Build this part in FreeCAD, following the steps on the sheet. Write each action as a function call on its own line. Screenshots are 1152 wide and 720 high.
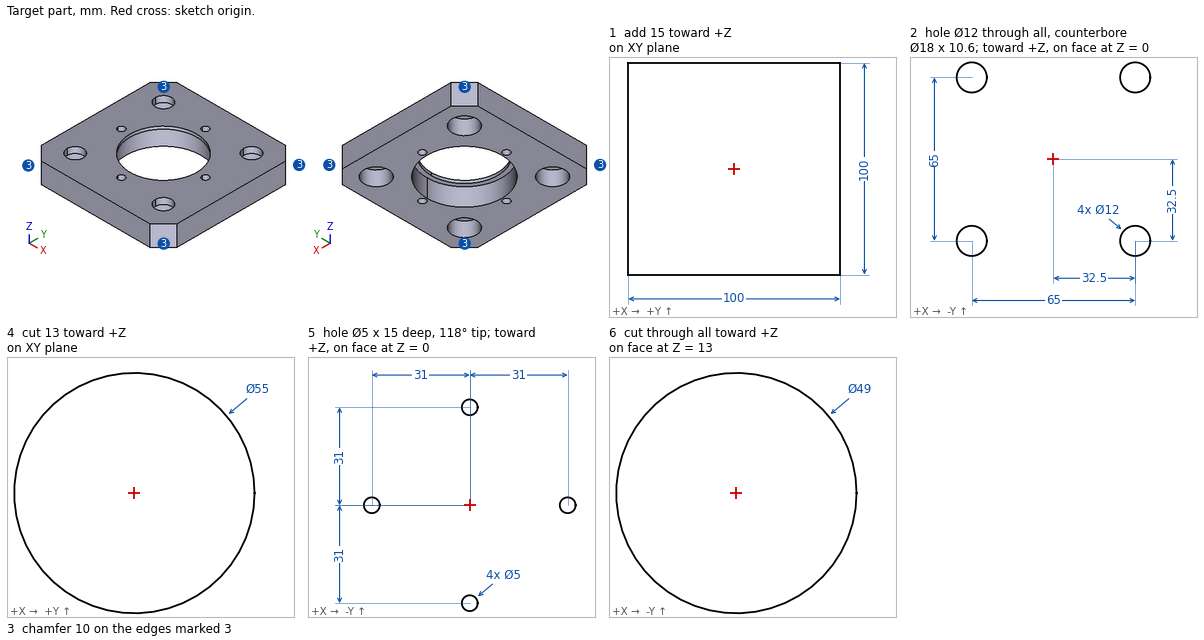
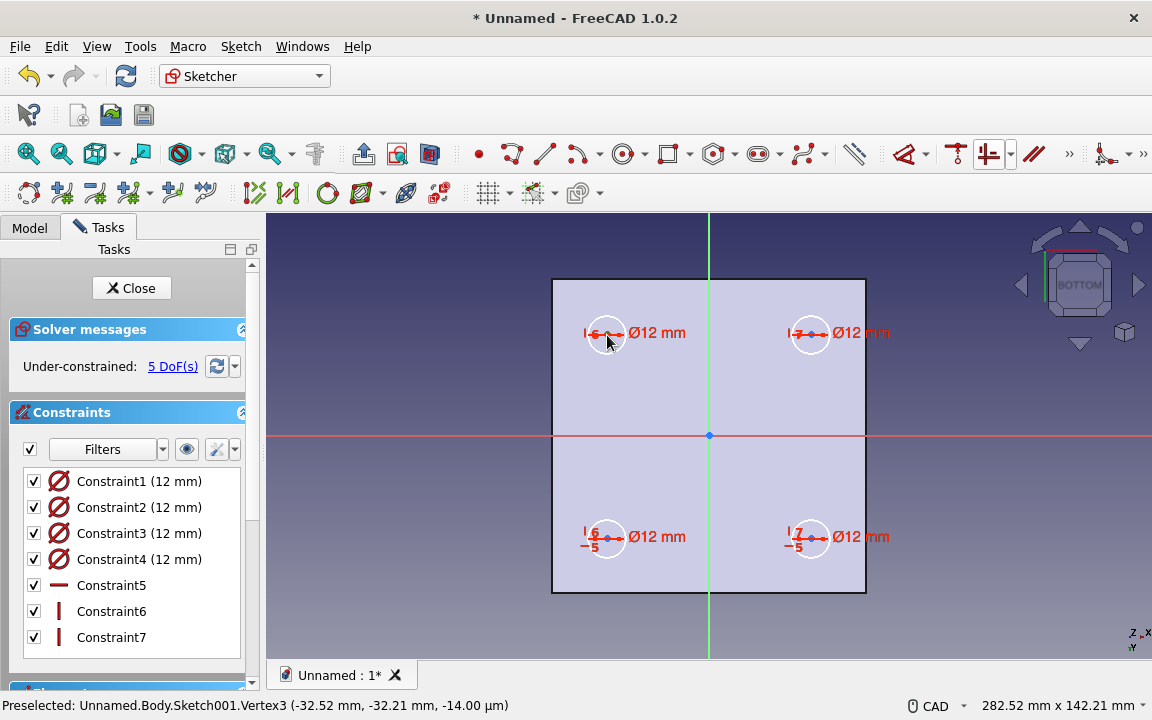
click(811, 335)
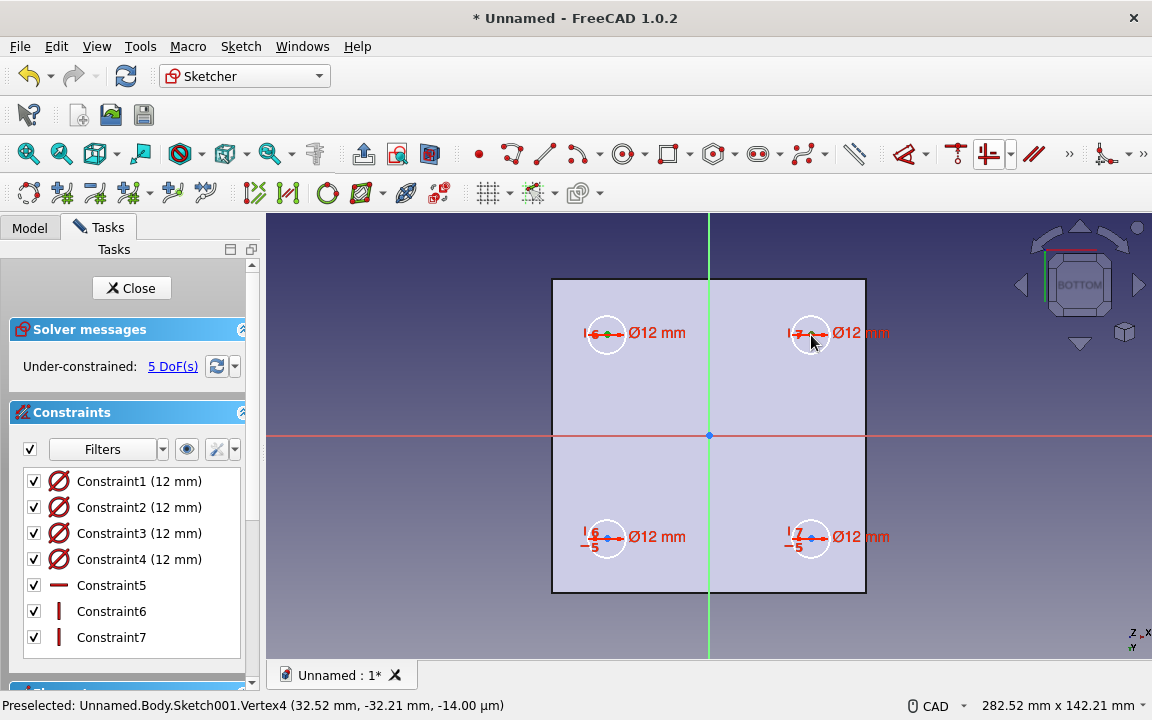
click(1010, 154)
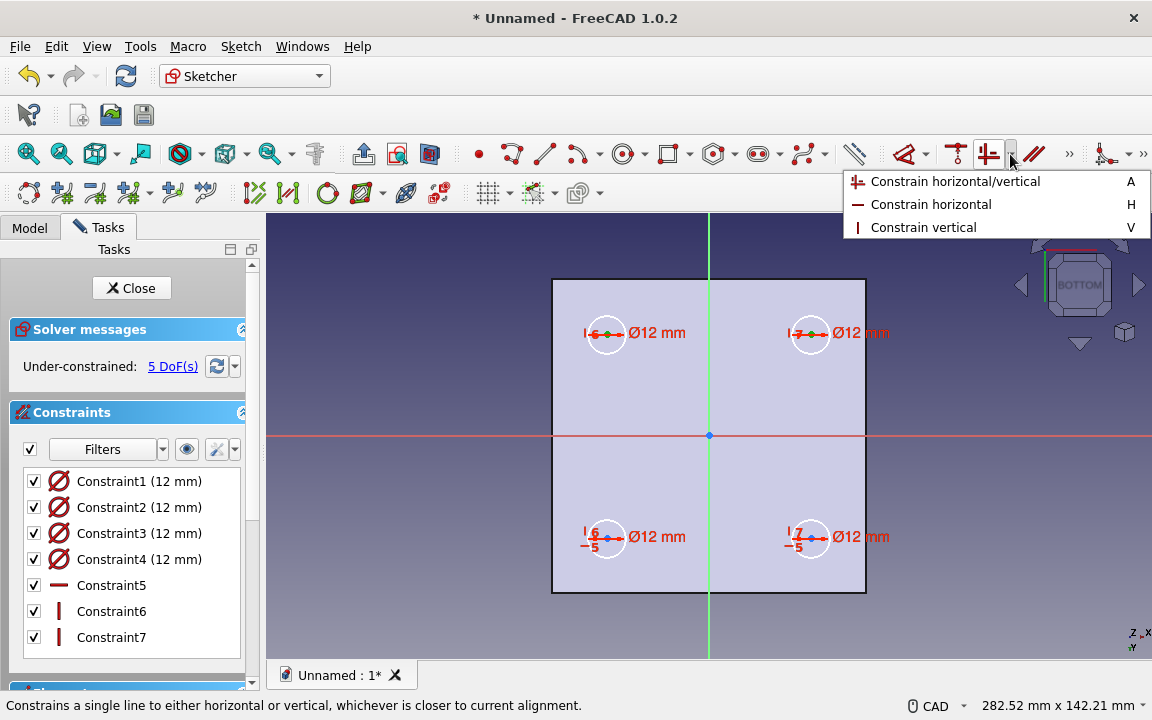
click(997, 204)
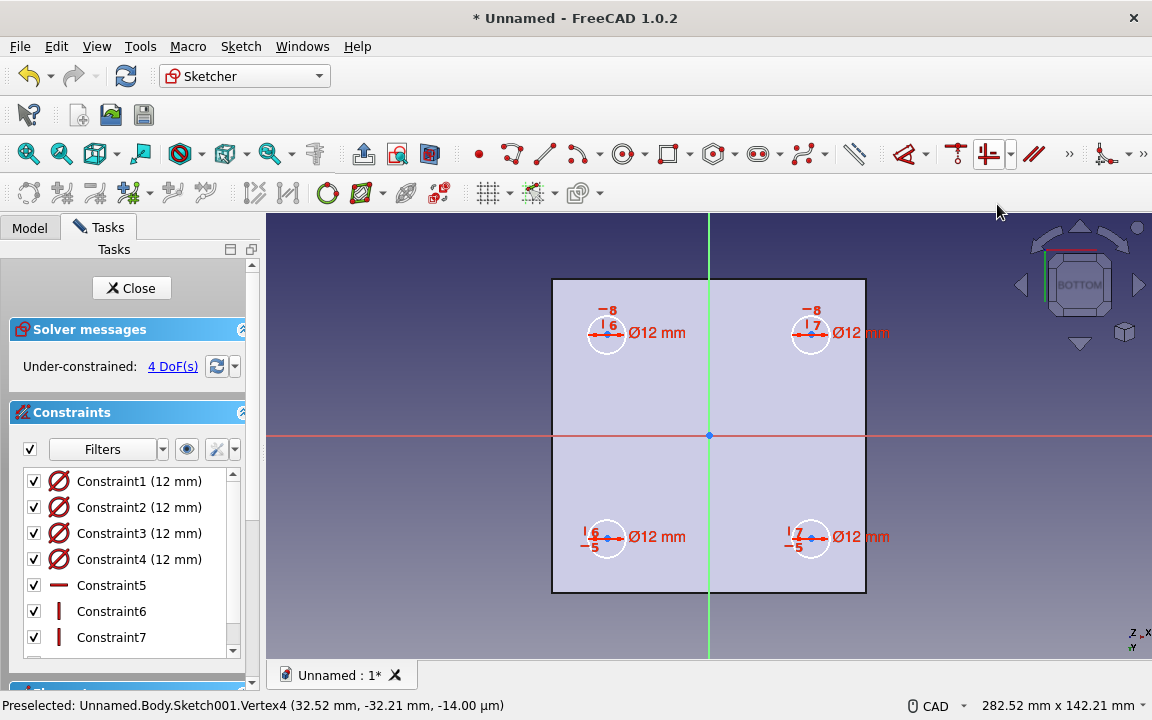
click(904, 154)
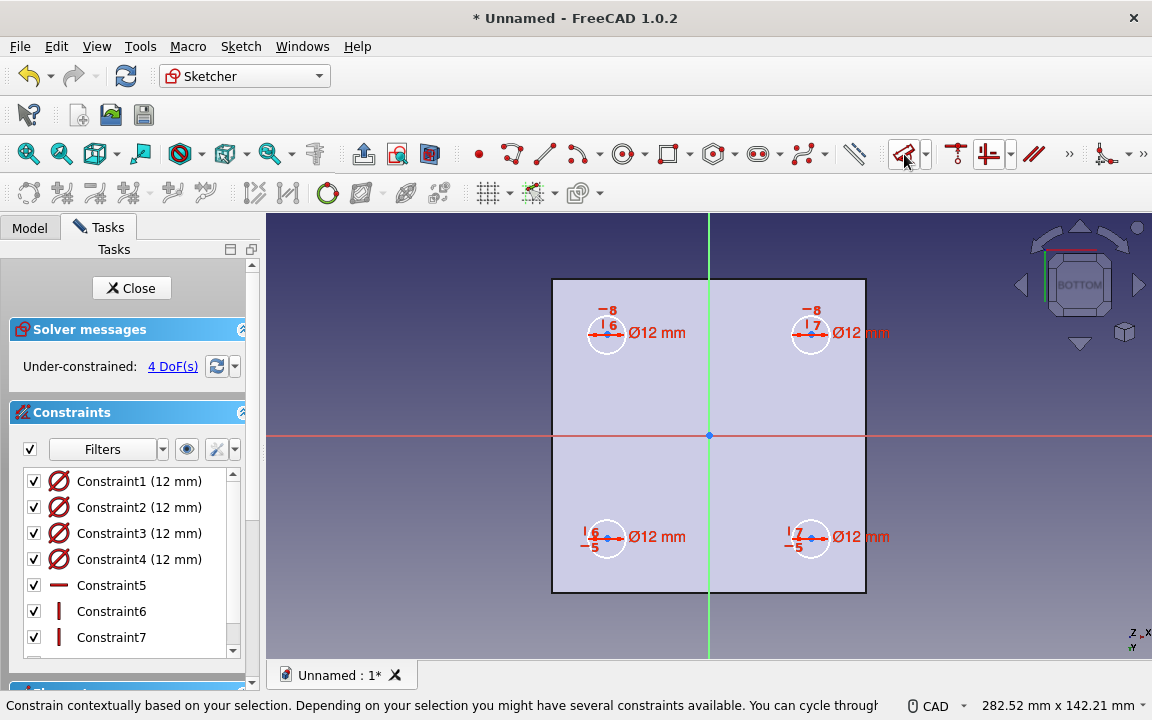
click(811, 539)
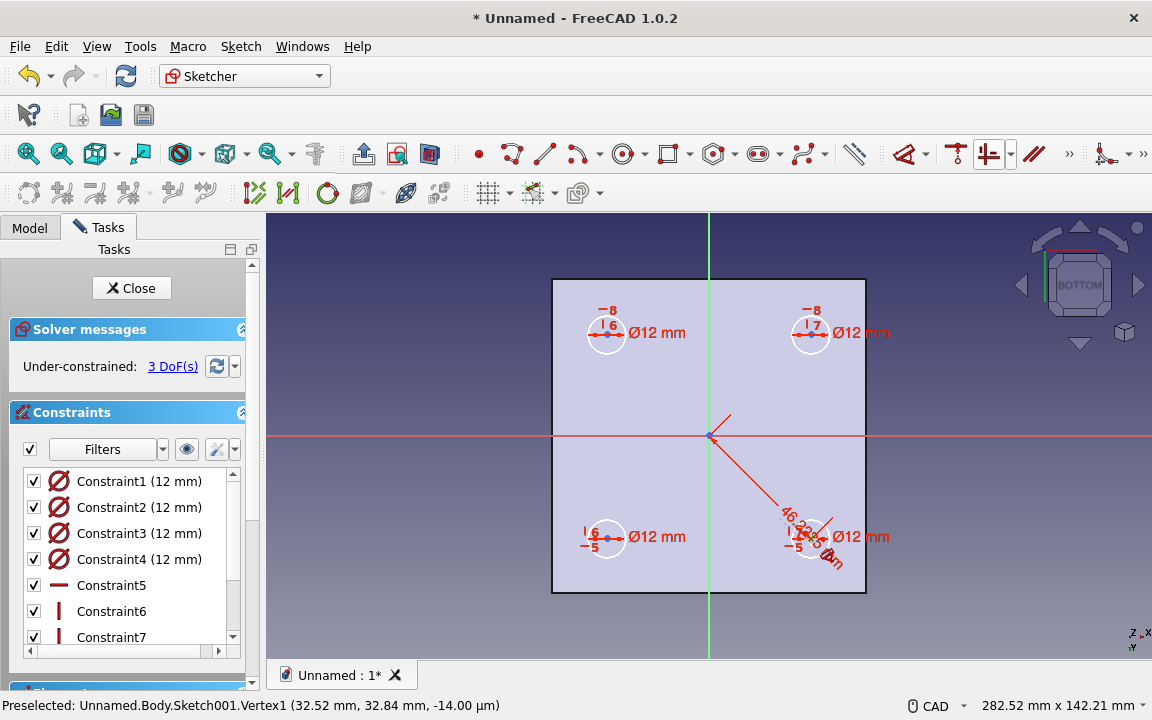
click(607, 539)
click(662, 573)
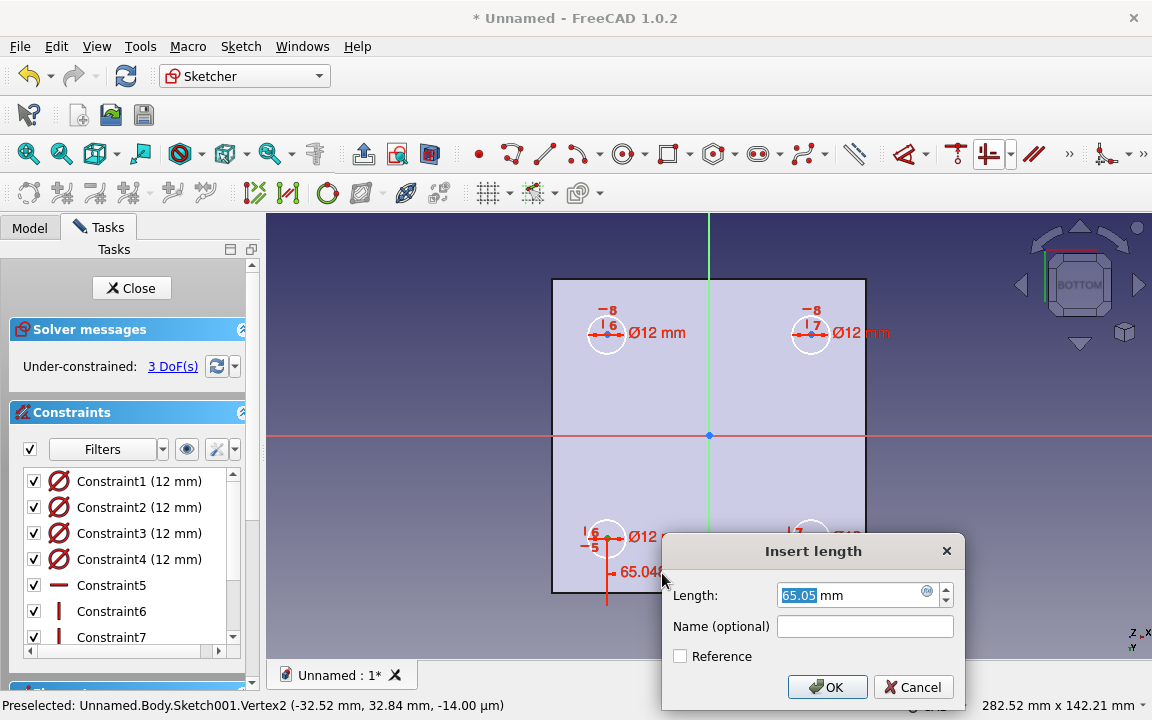
text(65)
key(Return)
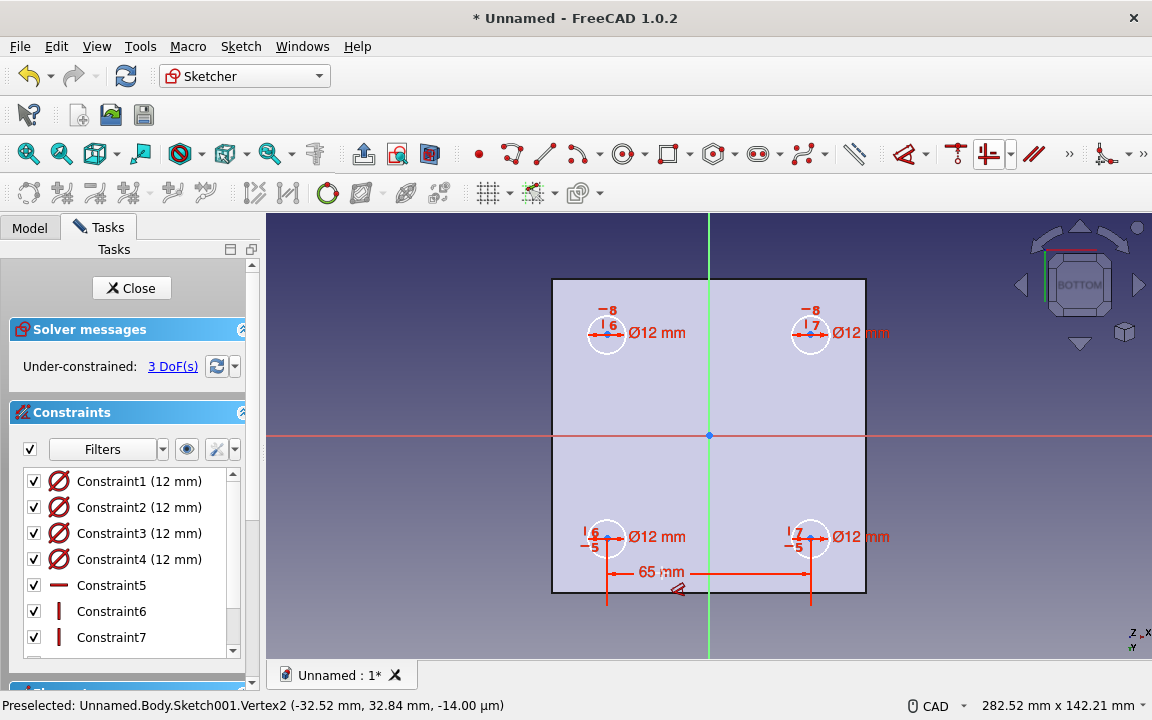
click(607, 539)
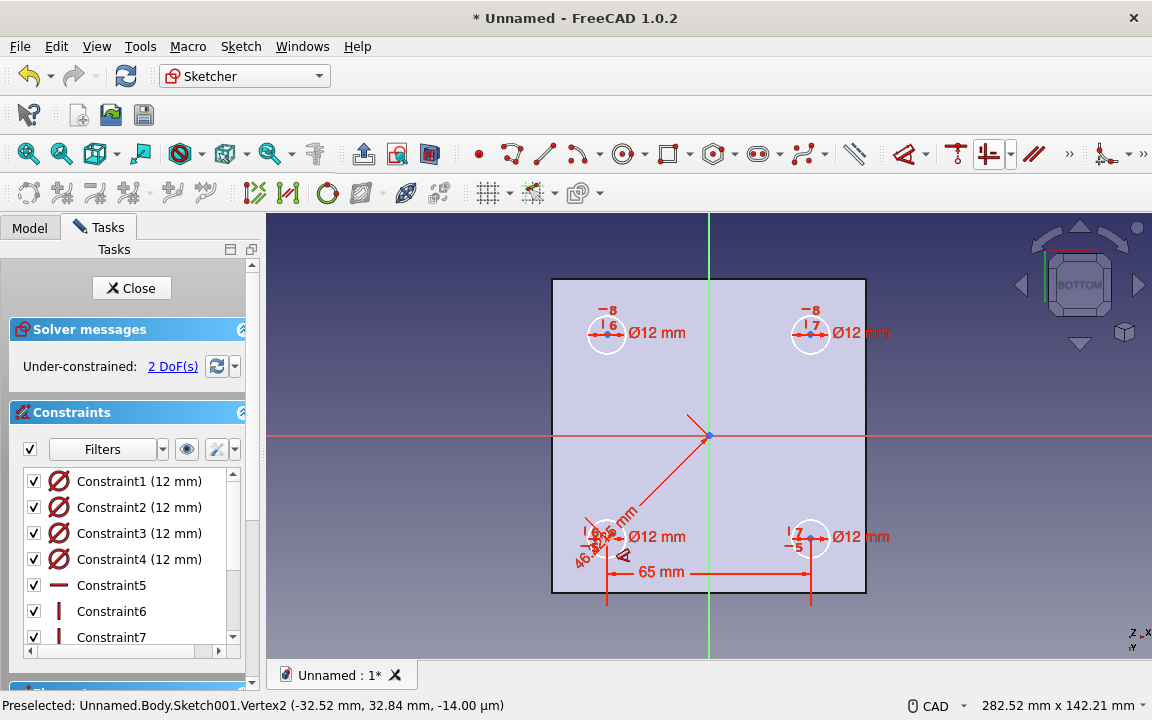
click(607, 335)
click(573, 390)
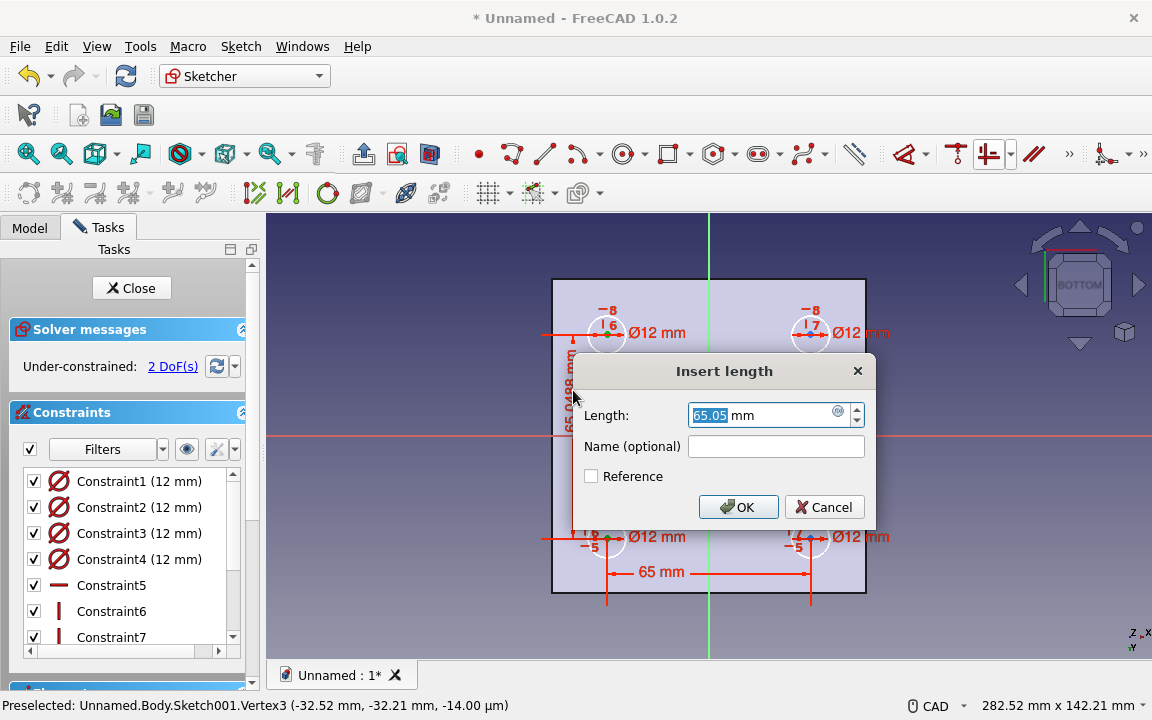
text(65)
key(Return)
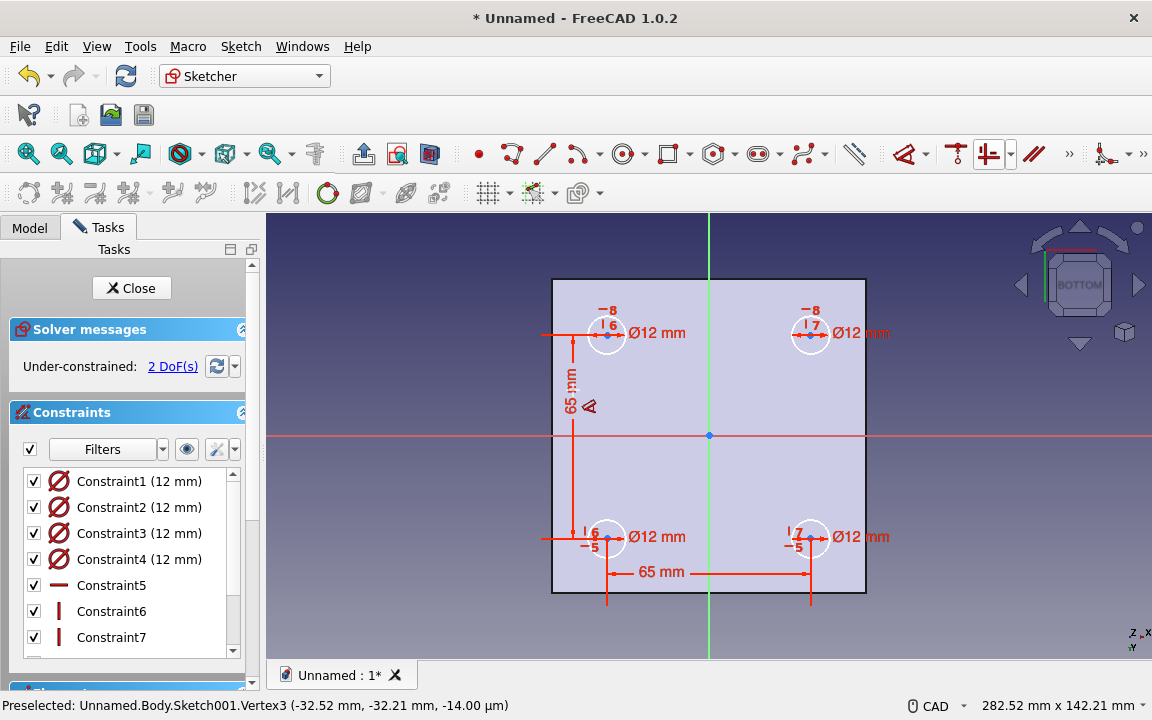
click(811, 539)
click(760, 573)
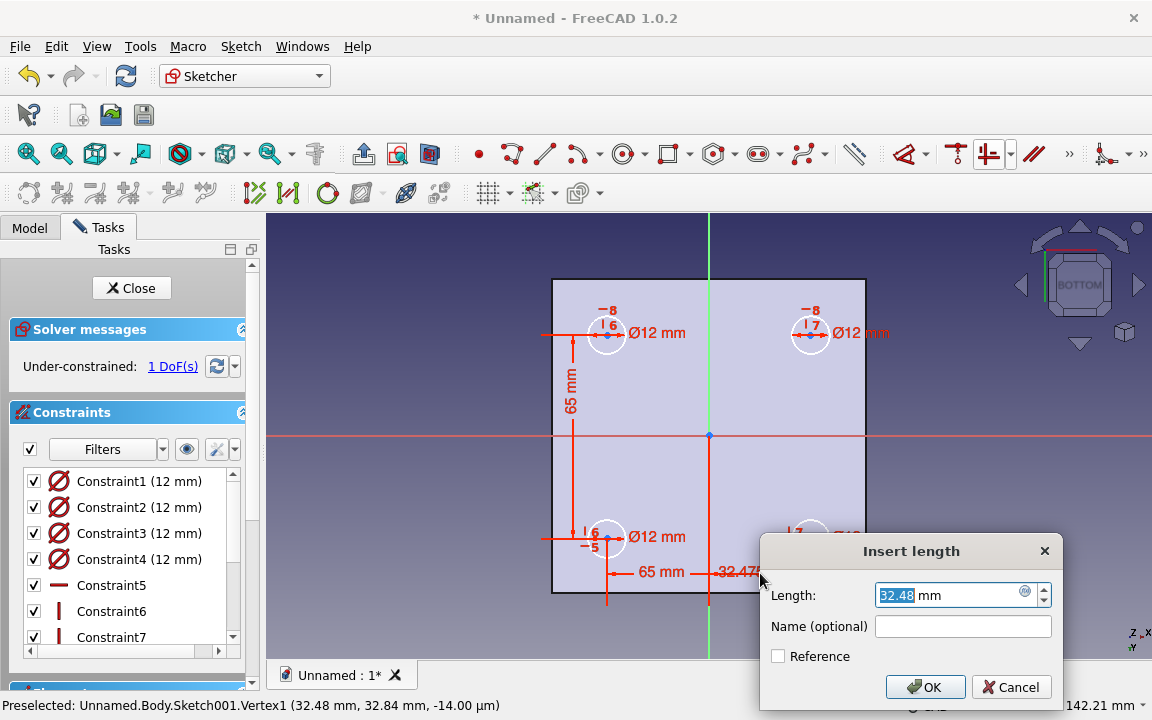
text(32.5)
key(Return)